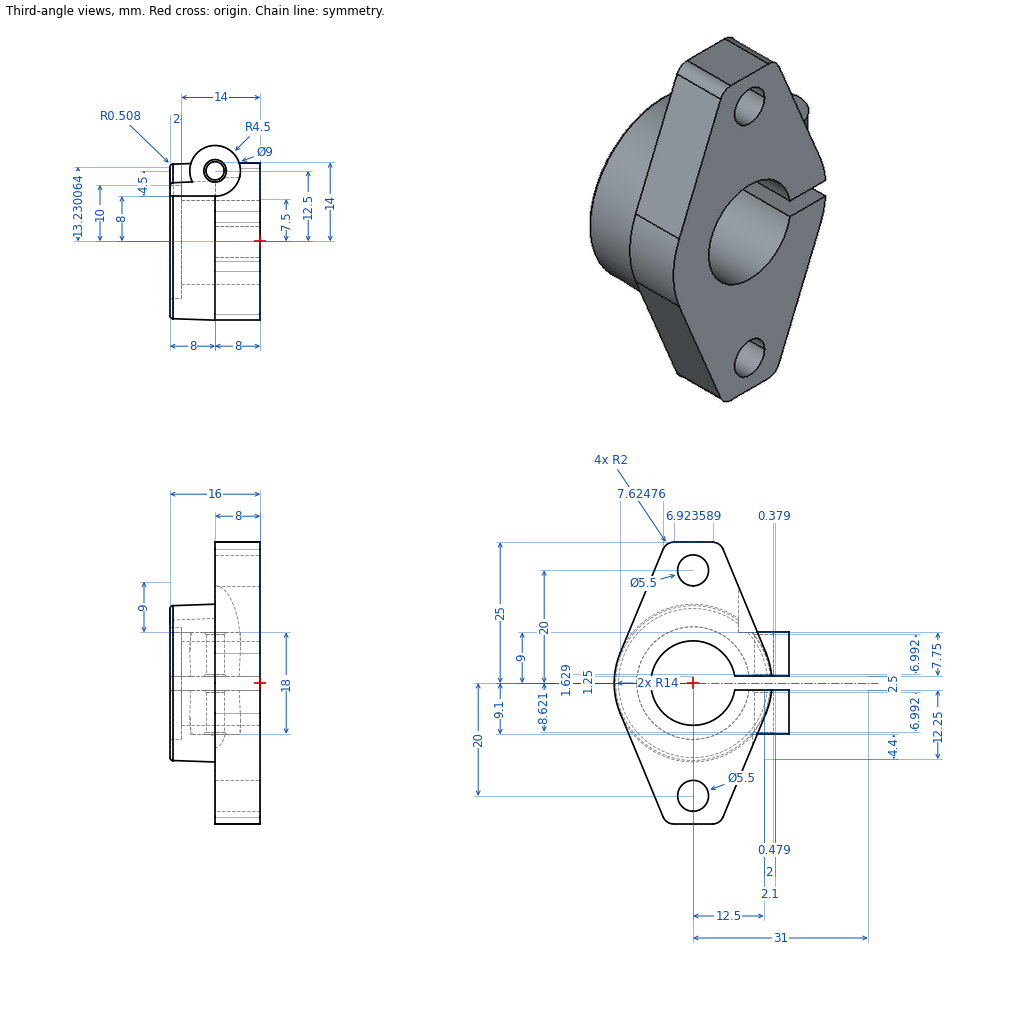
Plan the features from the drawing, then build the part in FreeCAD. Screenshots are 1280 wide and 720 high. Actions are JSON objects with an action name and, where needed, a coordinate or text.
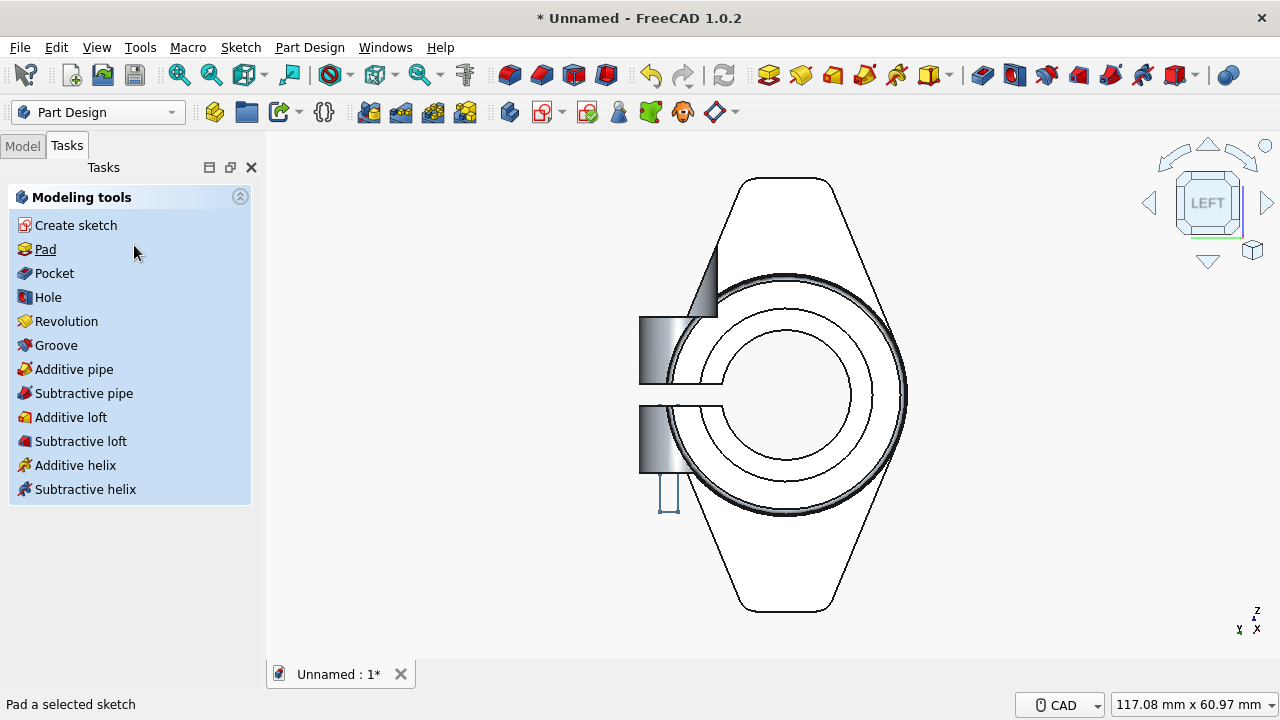
{"action": "left_click", "coordinate": [1048, 76]}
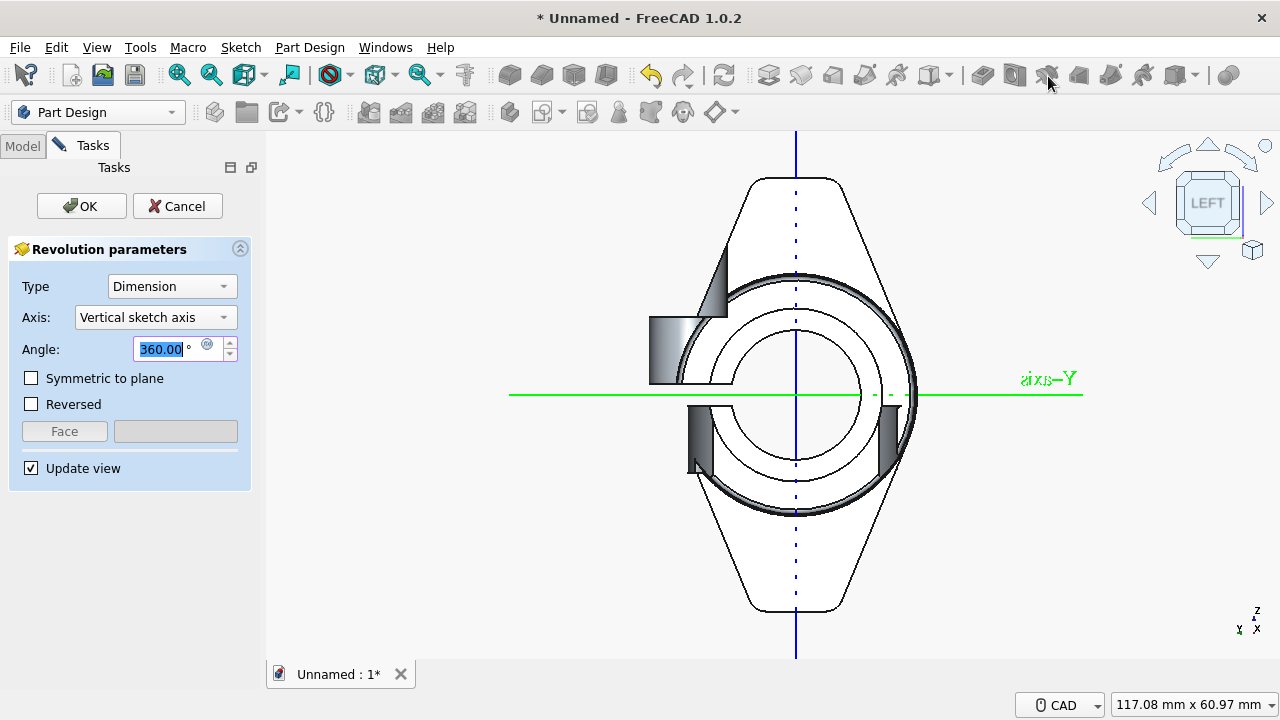
{"action": "left_click", "coordinate": [156, 318]}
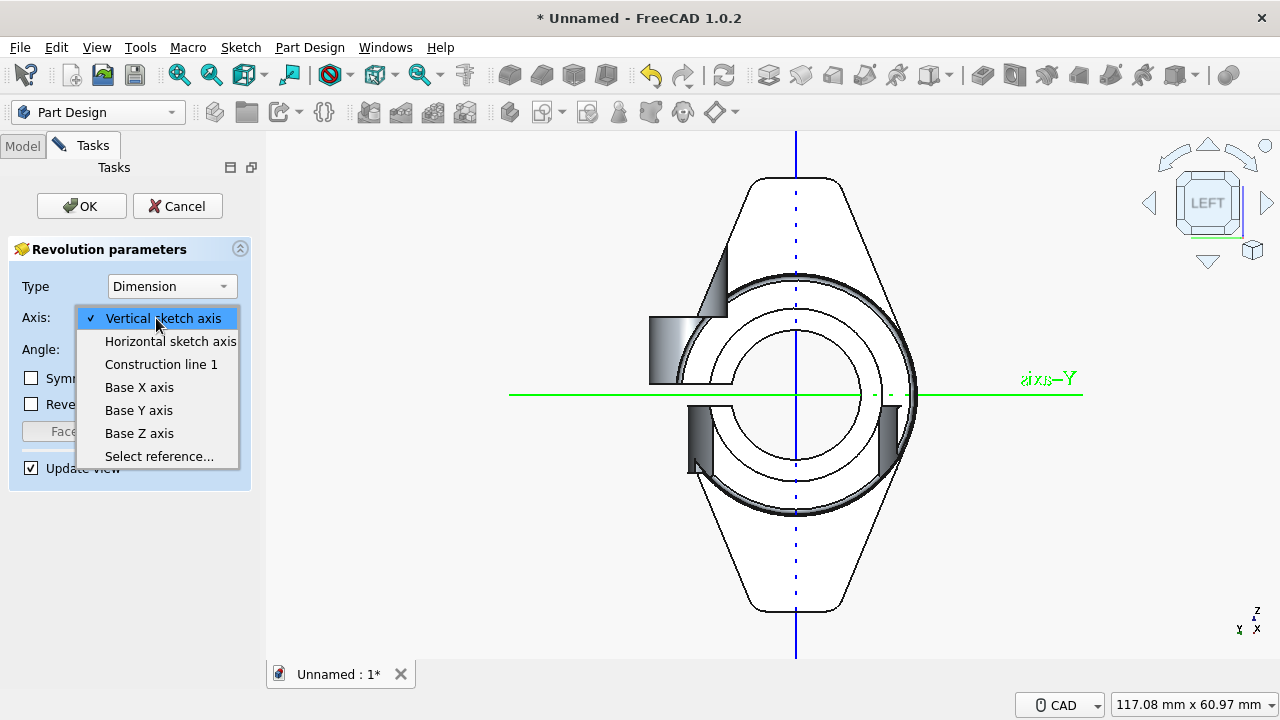
{"action": "left_click", "coordinate": [156, 364]}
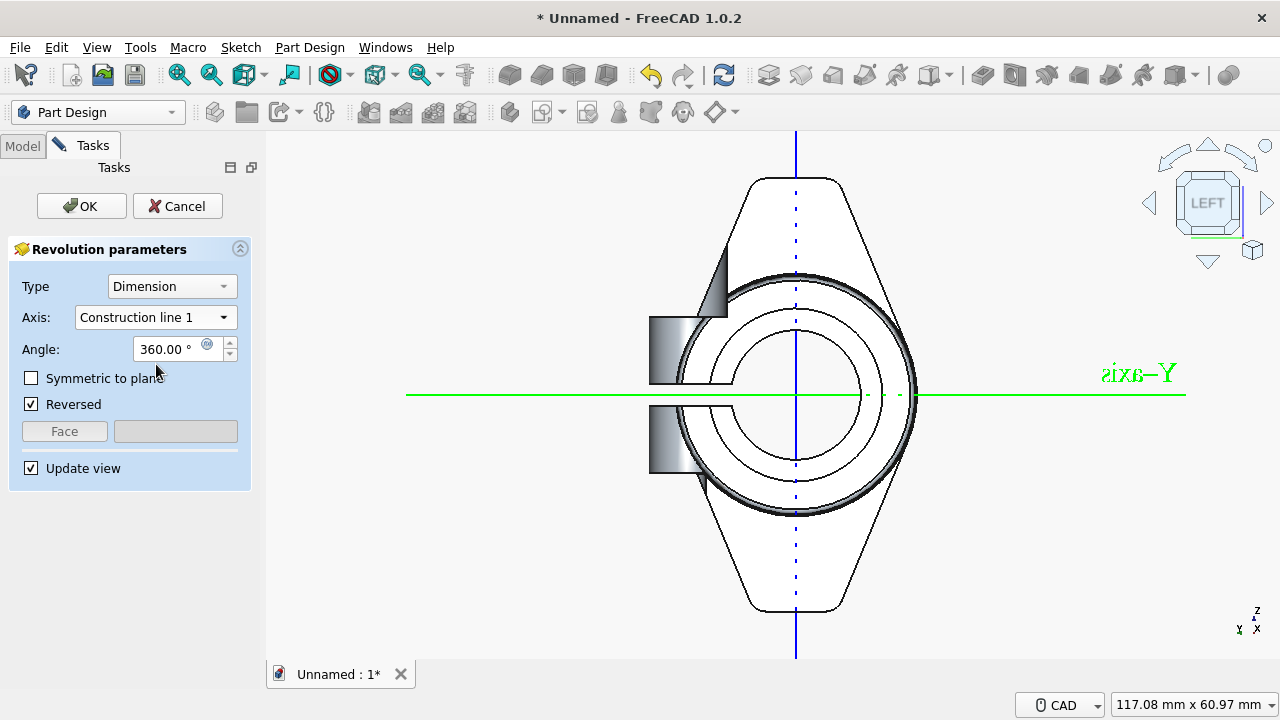
{"action": "left_click", "coordinate": [82, 206]}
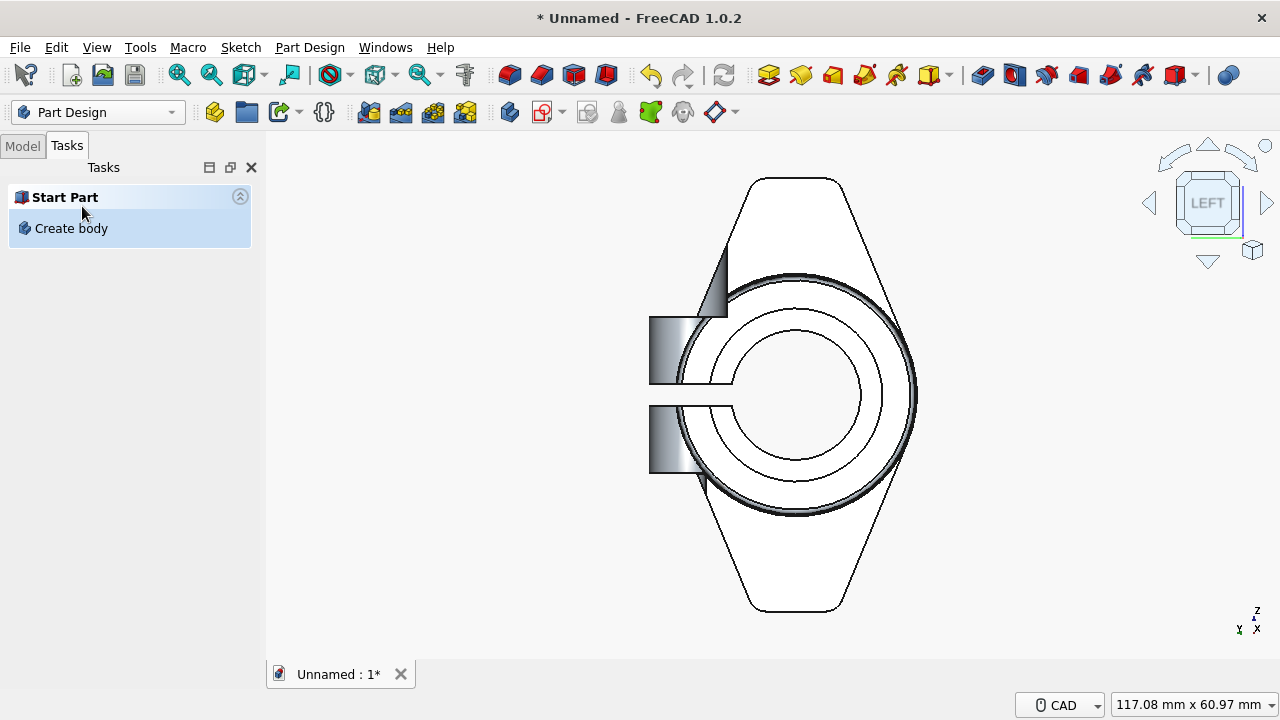
{"action": "left_click", "coordinate": [807, 574]}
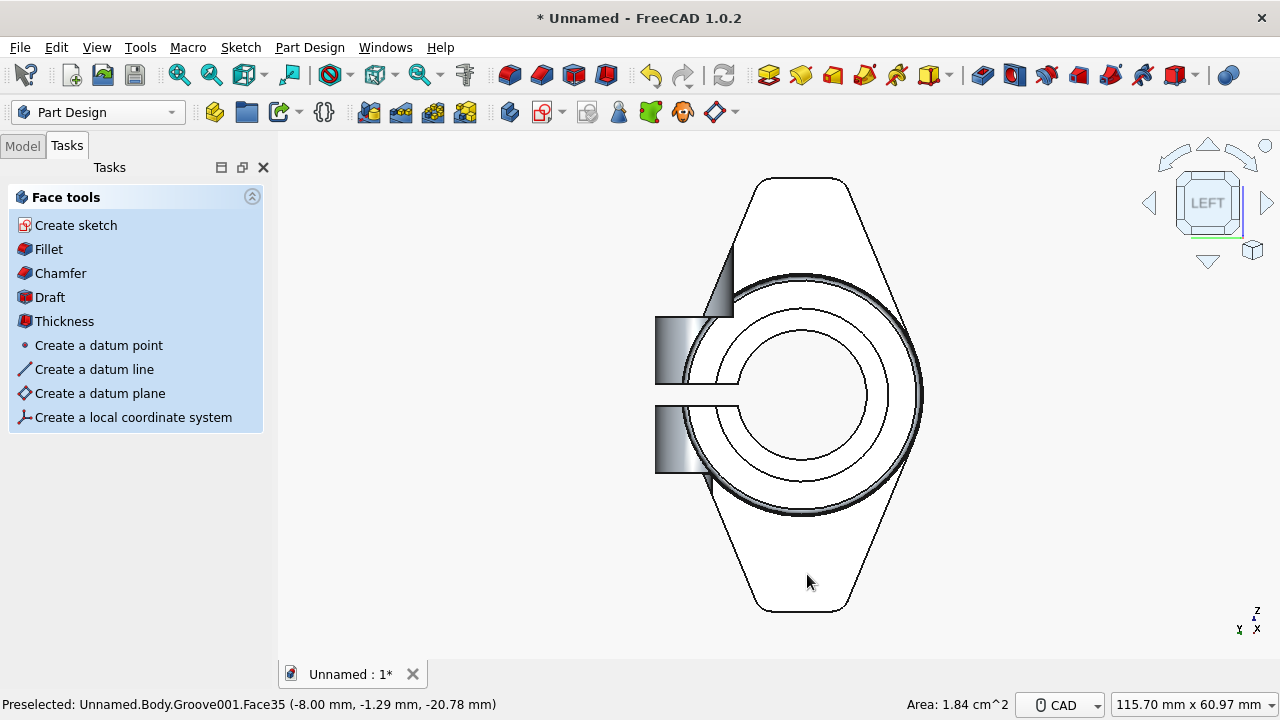
{"action": "left_click", "coordinate": [542, 112]}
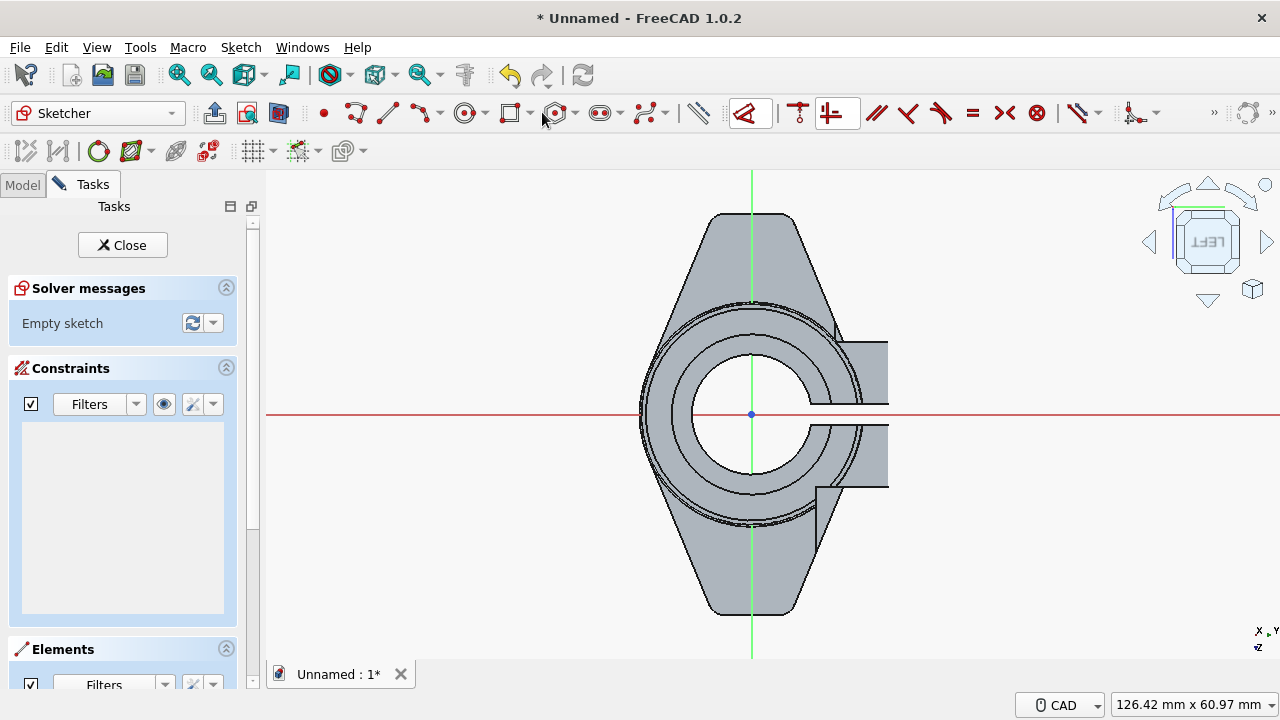
{"action": "scroll", "coordinate": [856, 484], "scroll_direction": "up", "scroll_amount": 6}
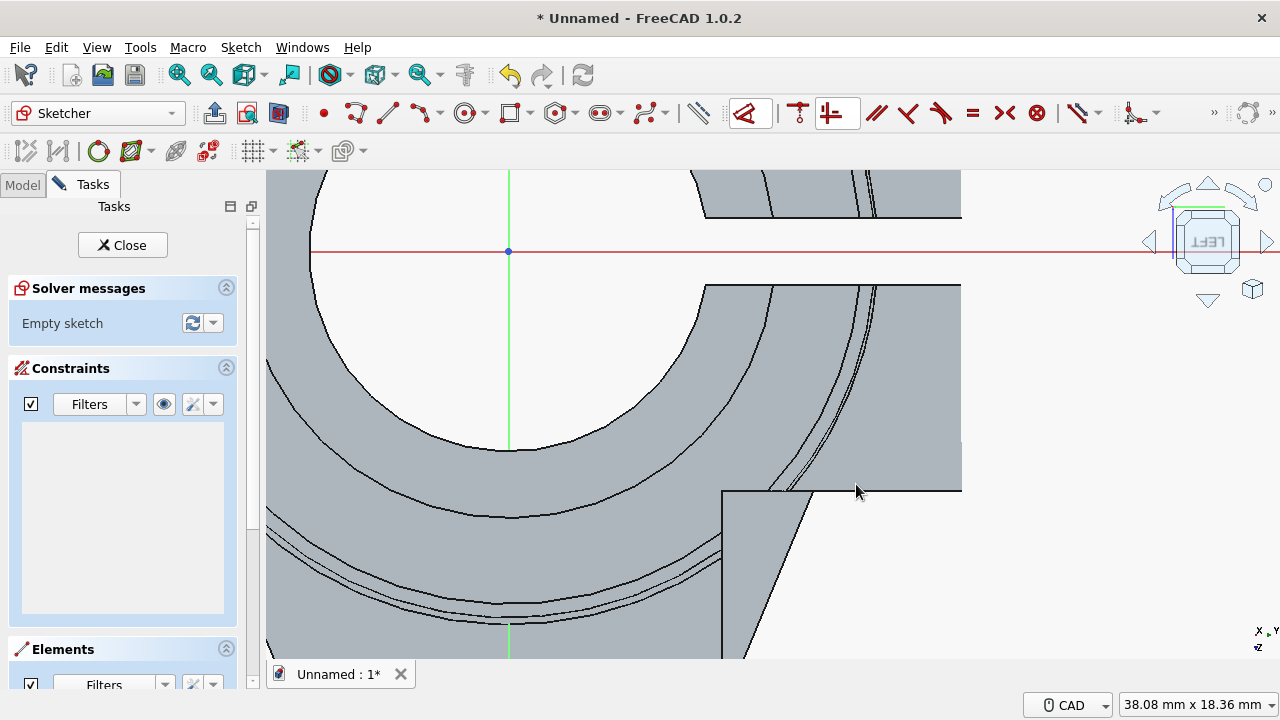
{"action": "left_click", "coordinate": [356, 114]}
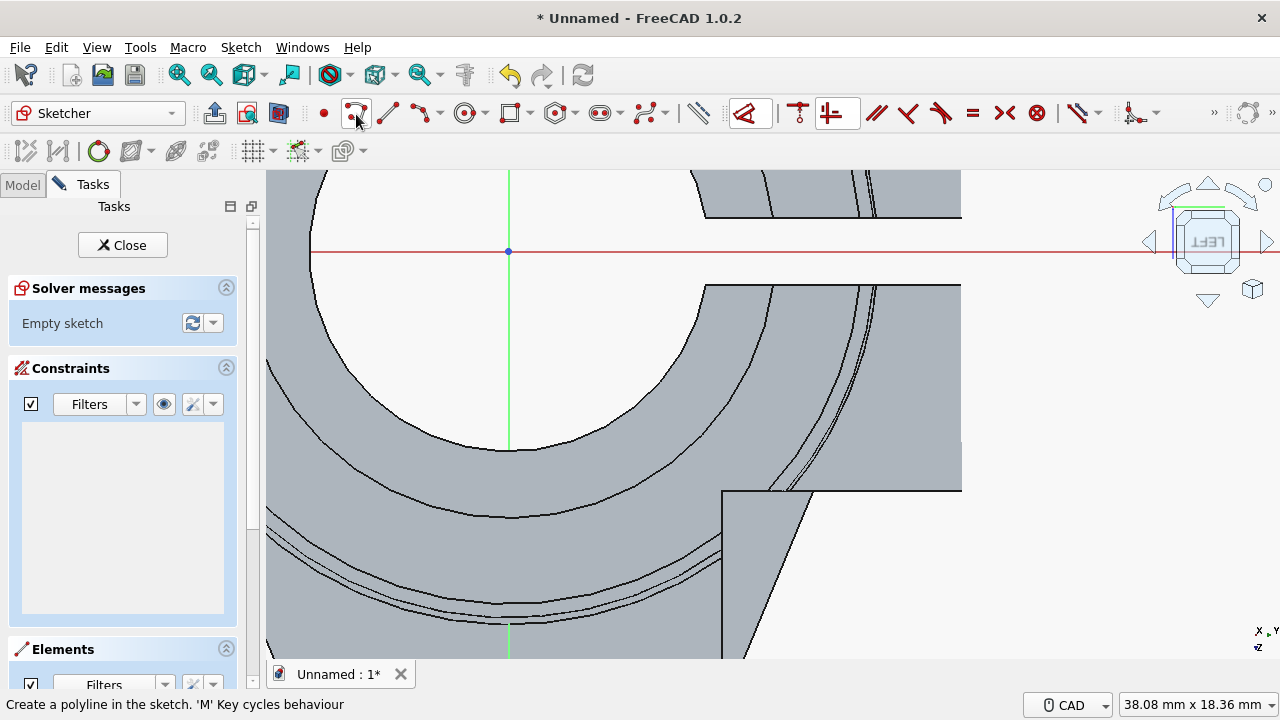
{"action": "left_click", "coordinate": [842, 285]}
{"action": "left_click", "coordinate": [895, 285]}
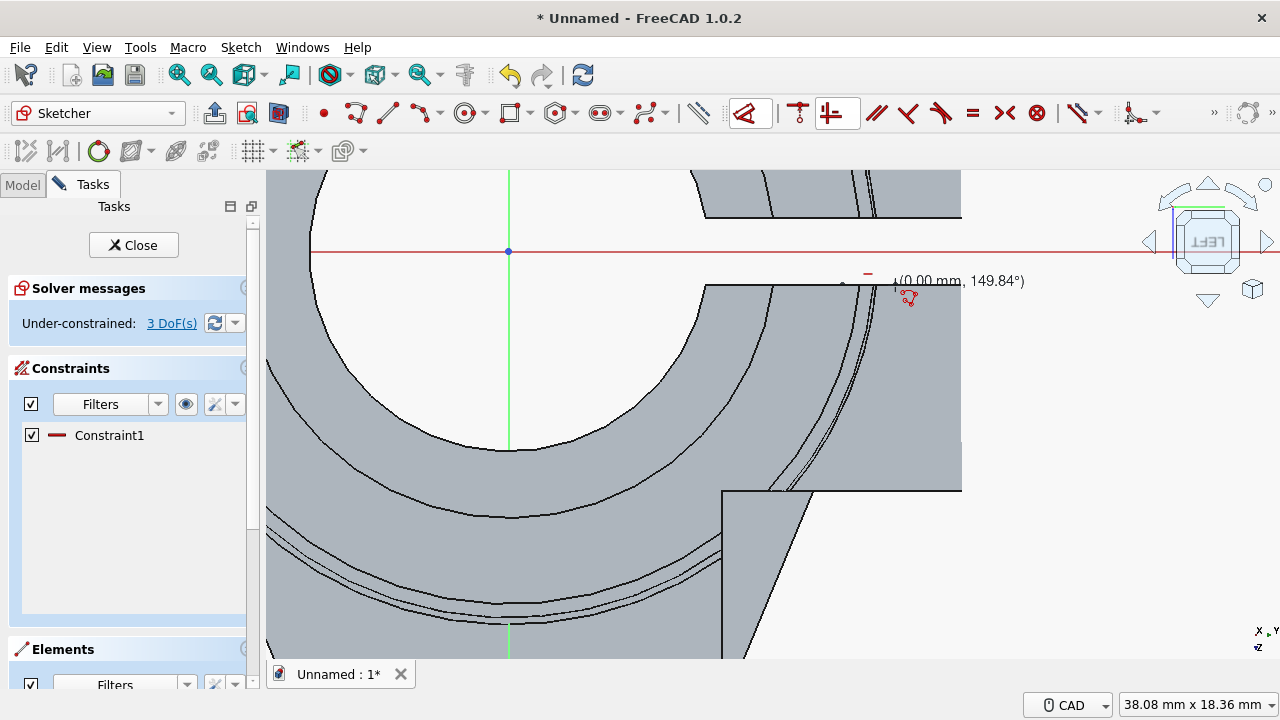
{"action": "scroll", "coordinate": [885, 295], "scroll_direction": "up", "scroll_amount": 3}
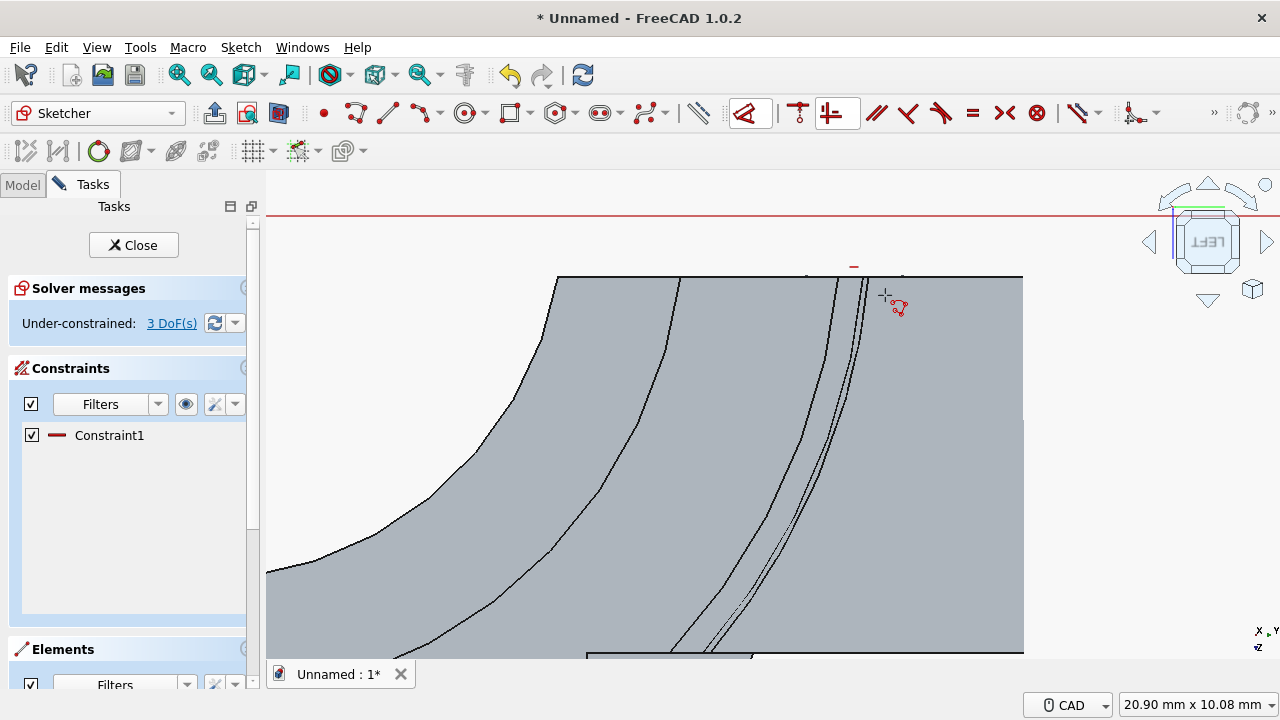
{"action": "left_click", "coordinate": [884, 295]}